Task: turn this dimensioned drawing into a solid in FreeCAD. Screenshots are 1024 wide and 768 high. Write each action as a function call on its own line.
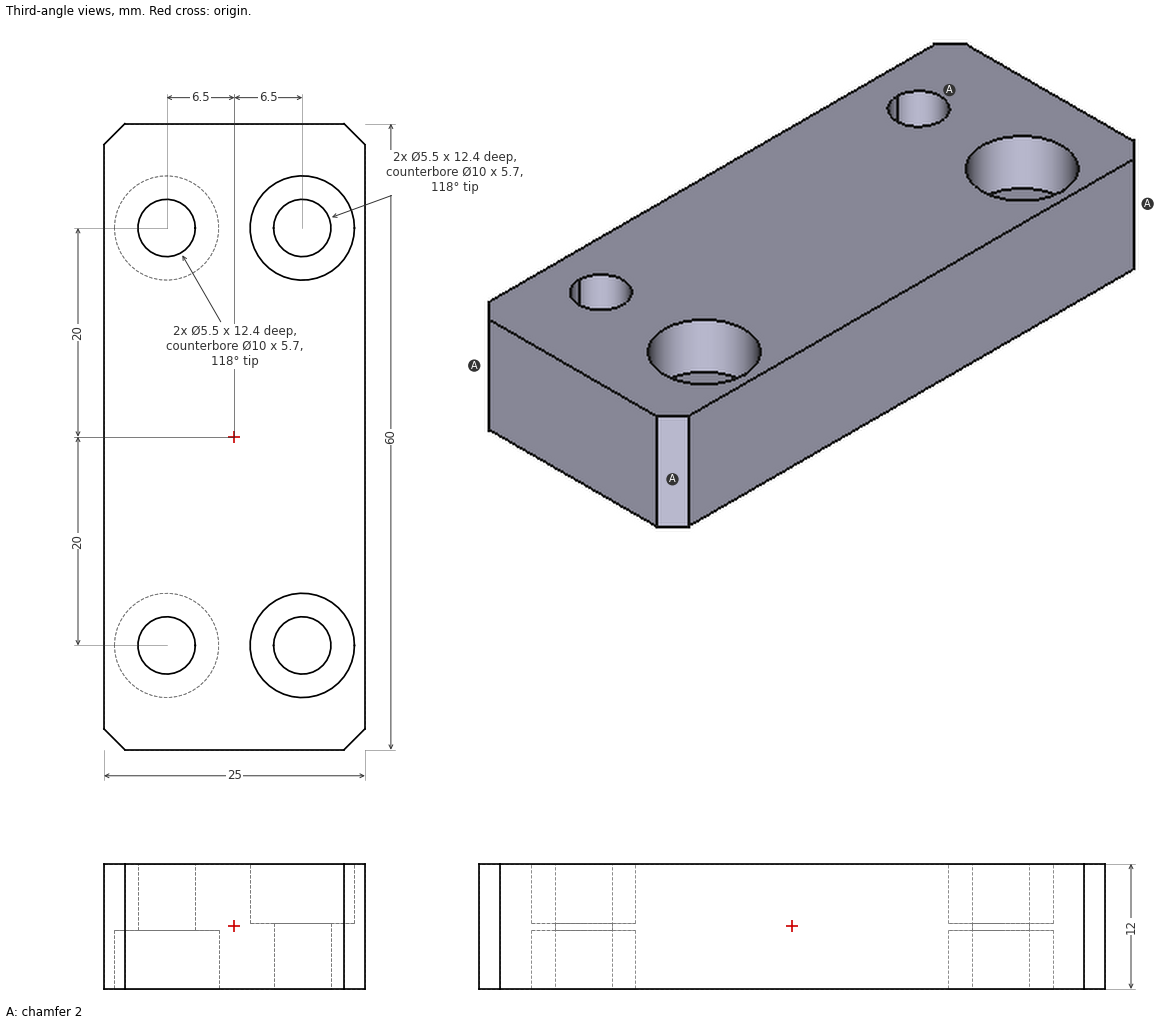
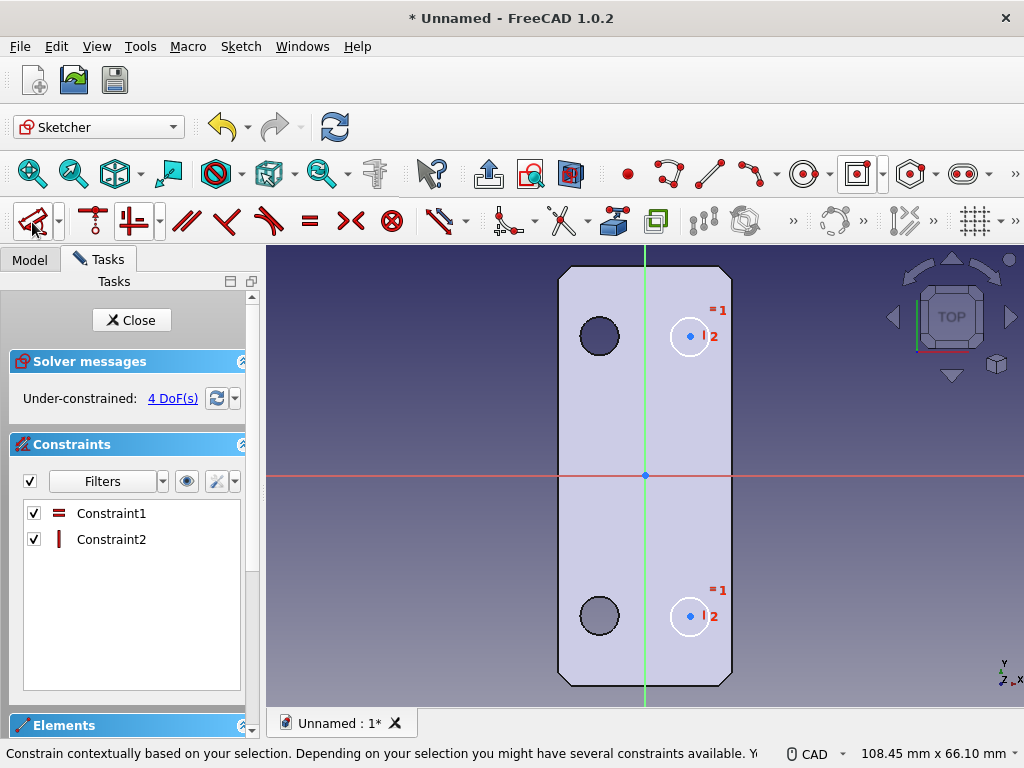
click(703, 323)
click(725, 300)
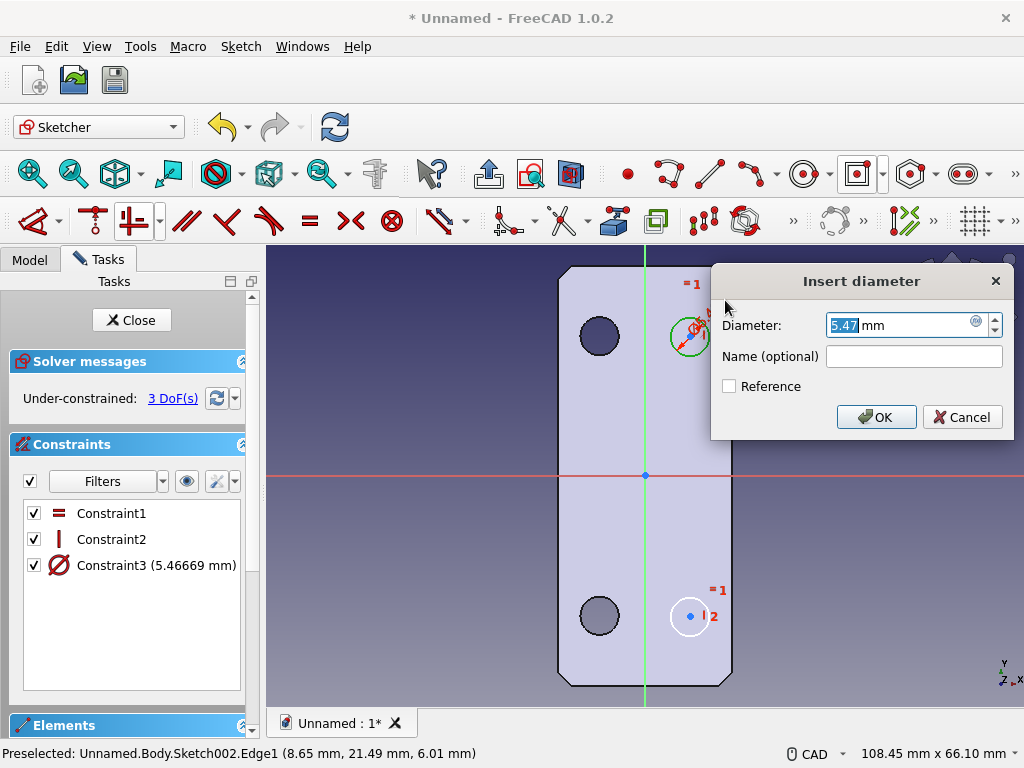
text(5.5)
key(Return)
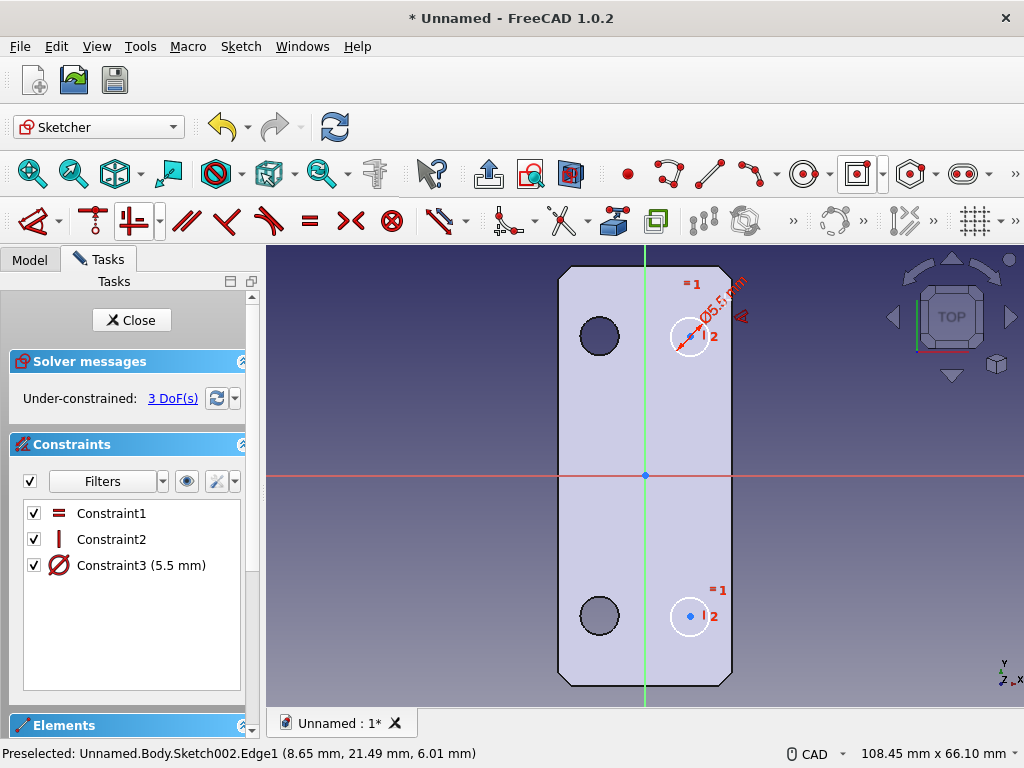
click(690, 337)
click(611, 406)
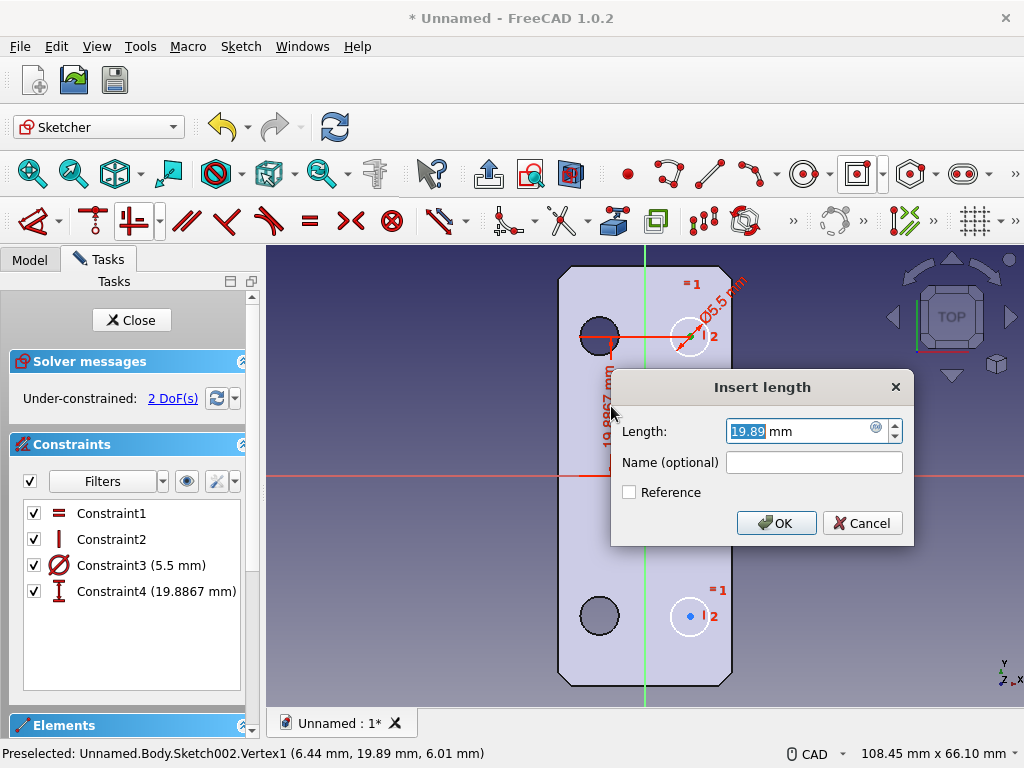
text(20)
key(Return)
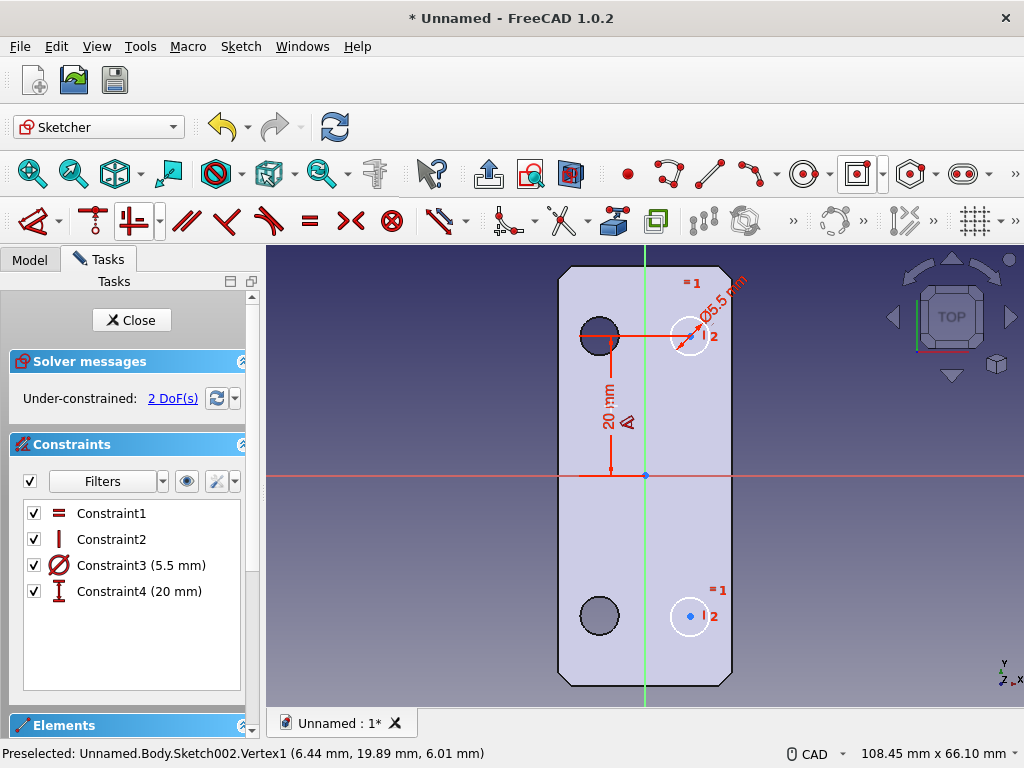
click(690, 617)
click(611, 546)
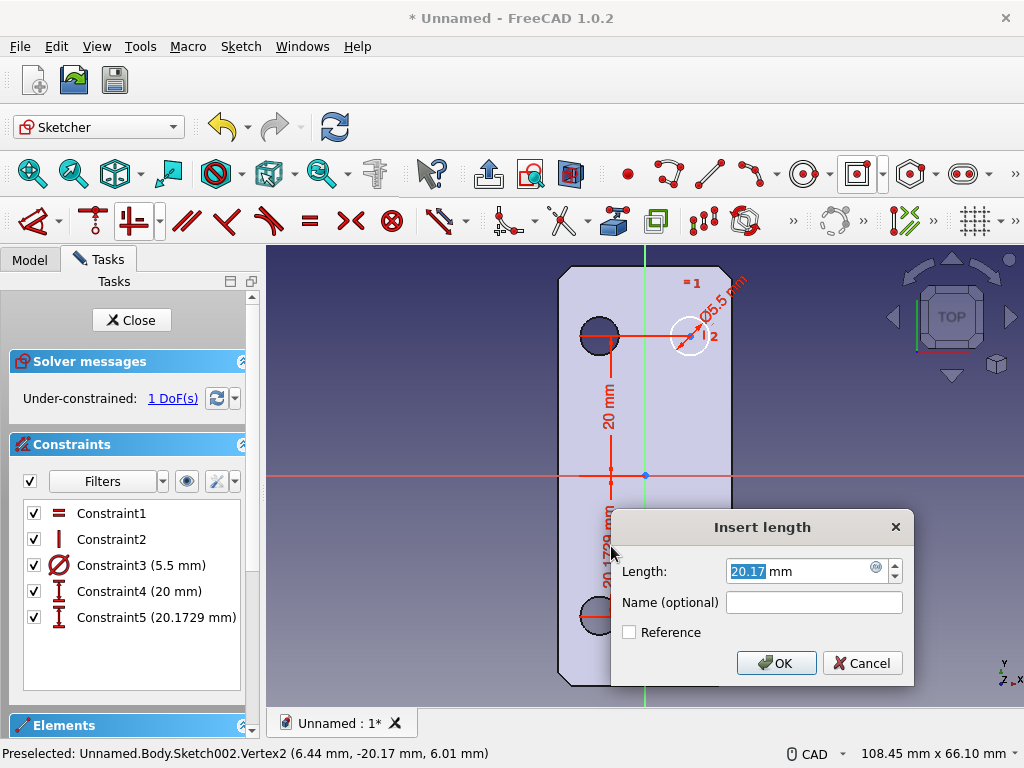
text(20)
key(Return)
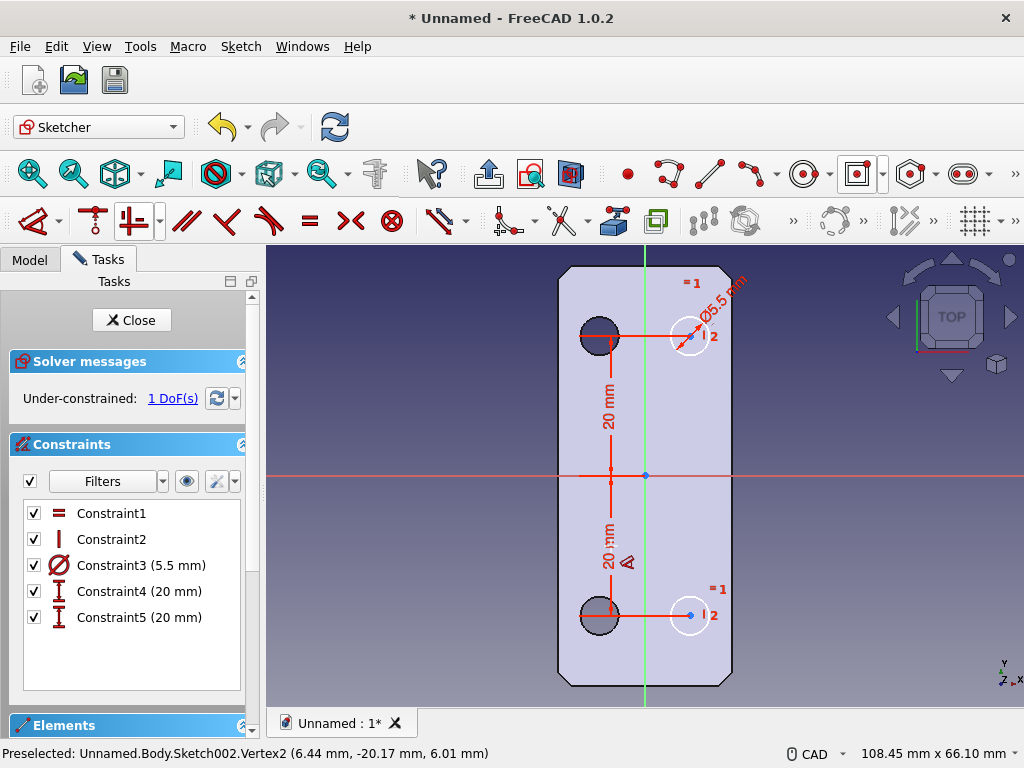
click(690, 336)
click(668, 510)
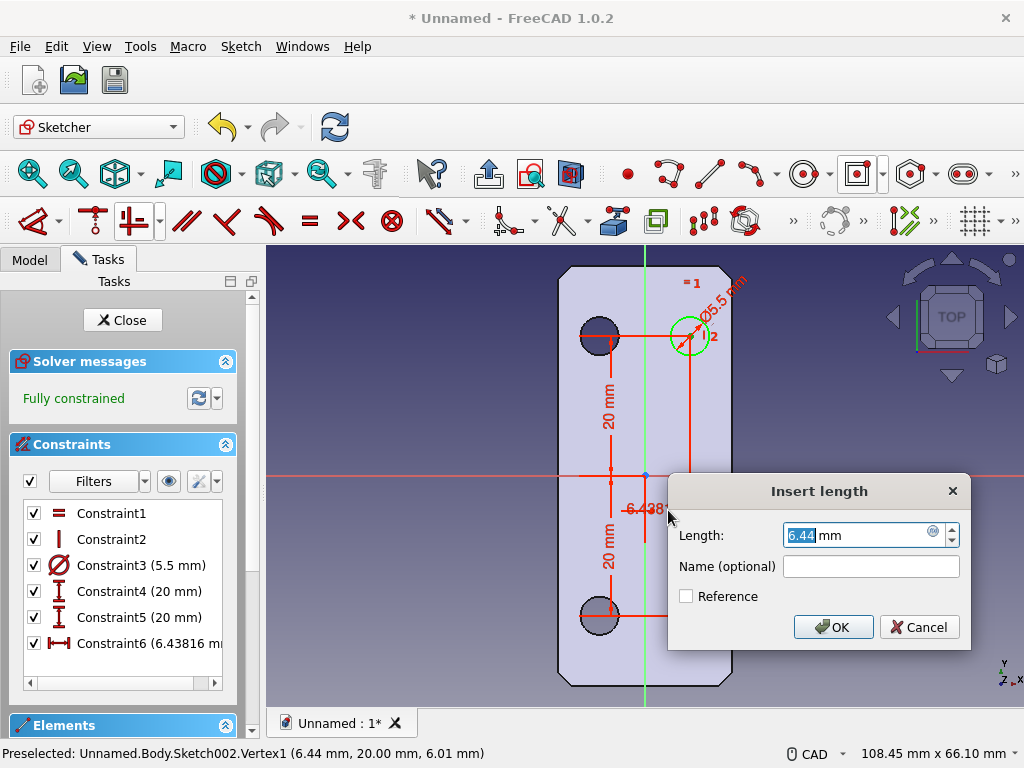
text(6.5)
key(Return)
key(Escape)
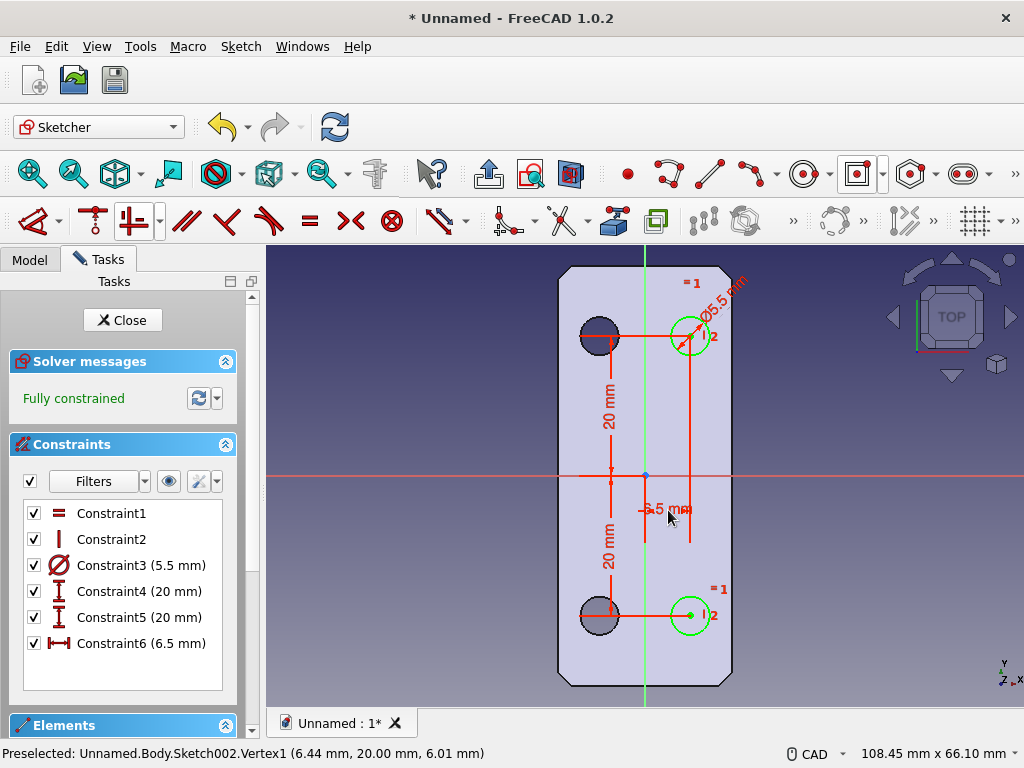
click(123, 320)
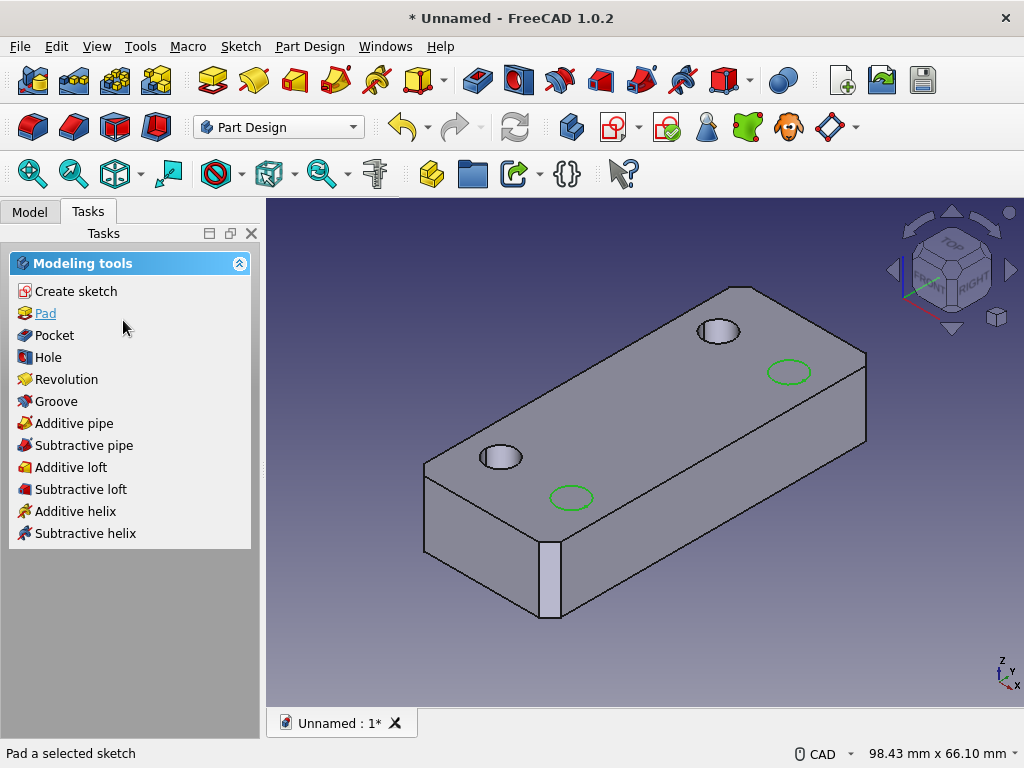
click(519, 80)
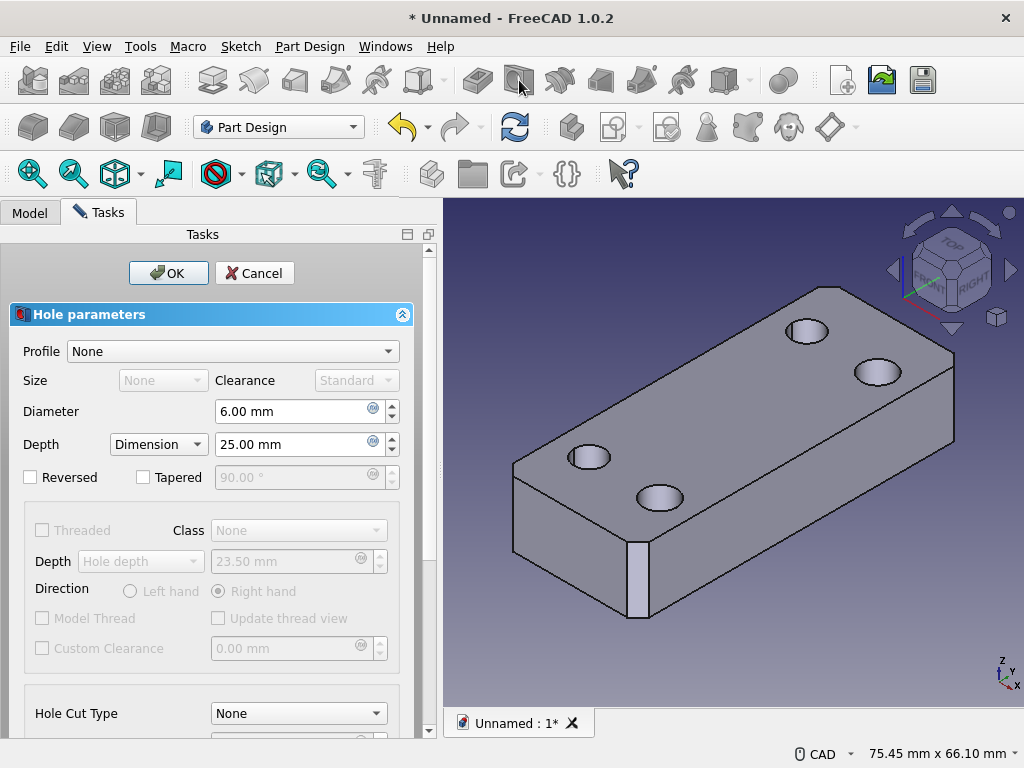
triple_click(300, 412)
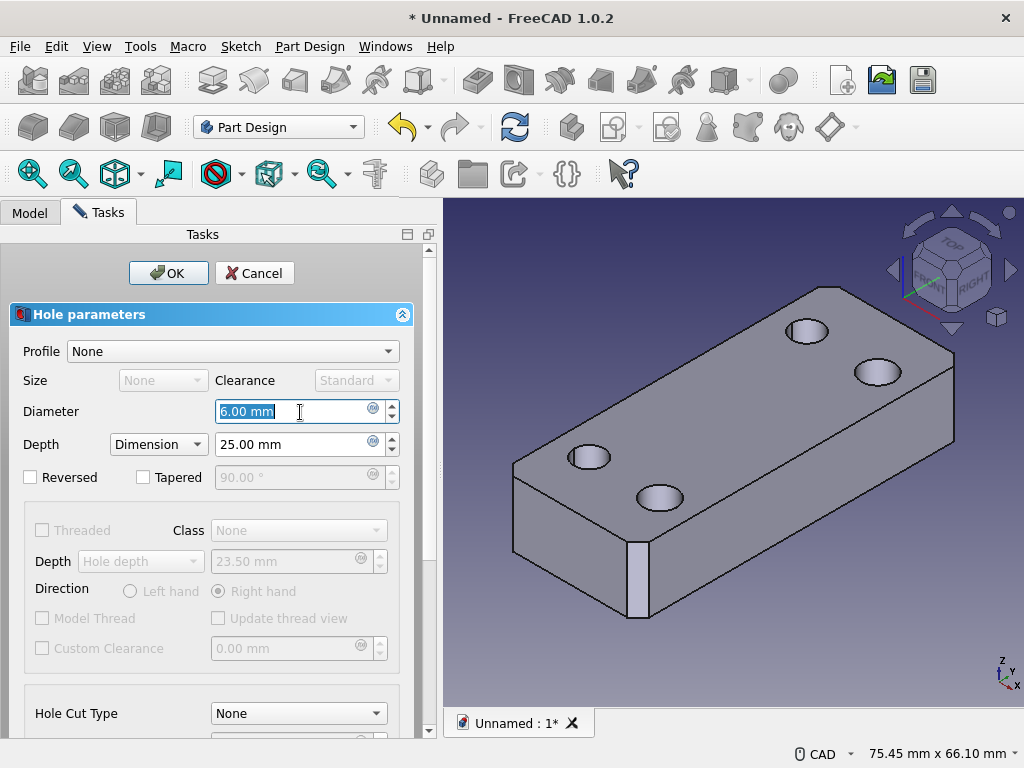
text(5.5)
key(Tab)